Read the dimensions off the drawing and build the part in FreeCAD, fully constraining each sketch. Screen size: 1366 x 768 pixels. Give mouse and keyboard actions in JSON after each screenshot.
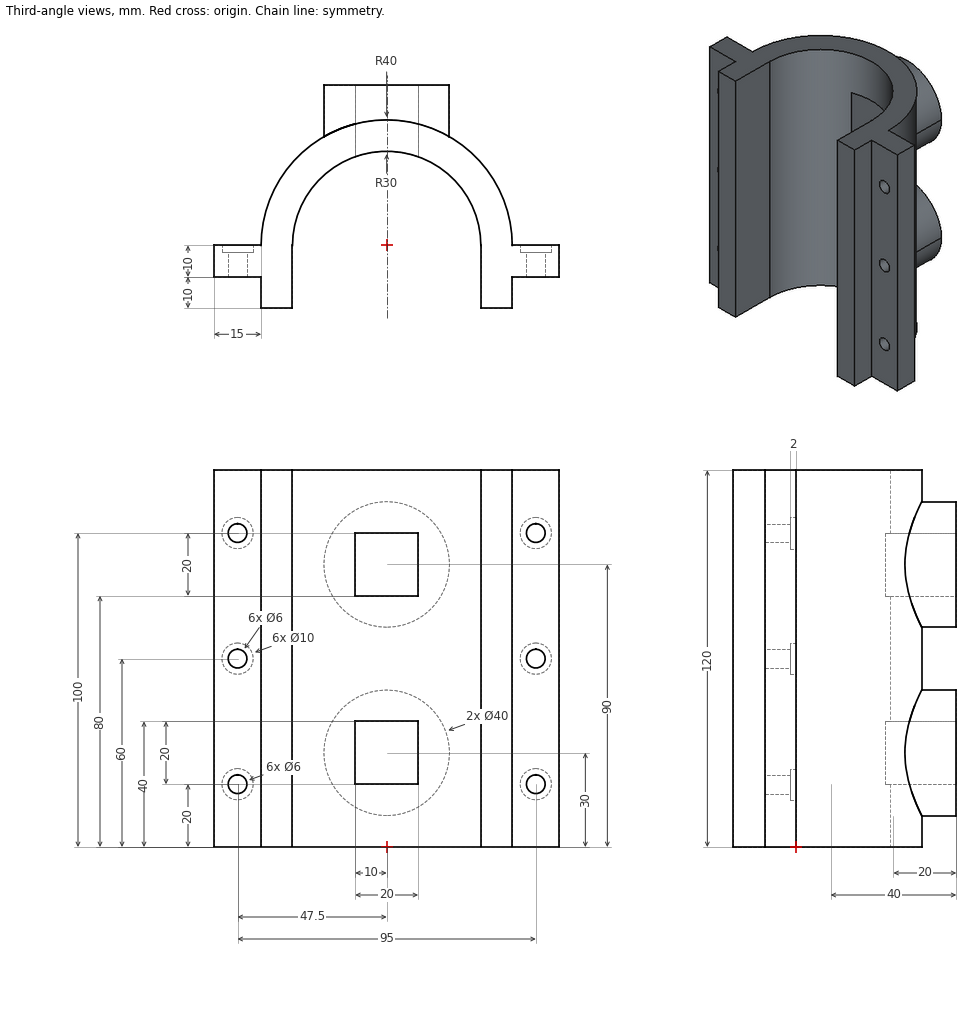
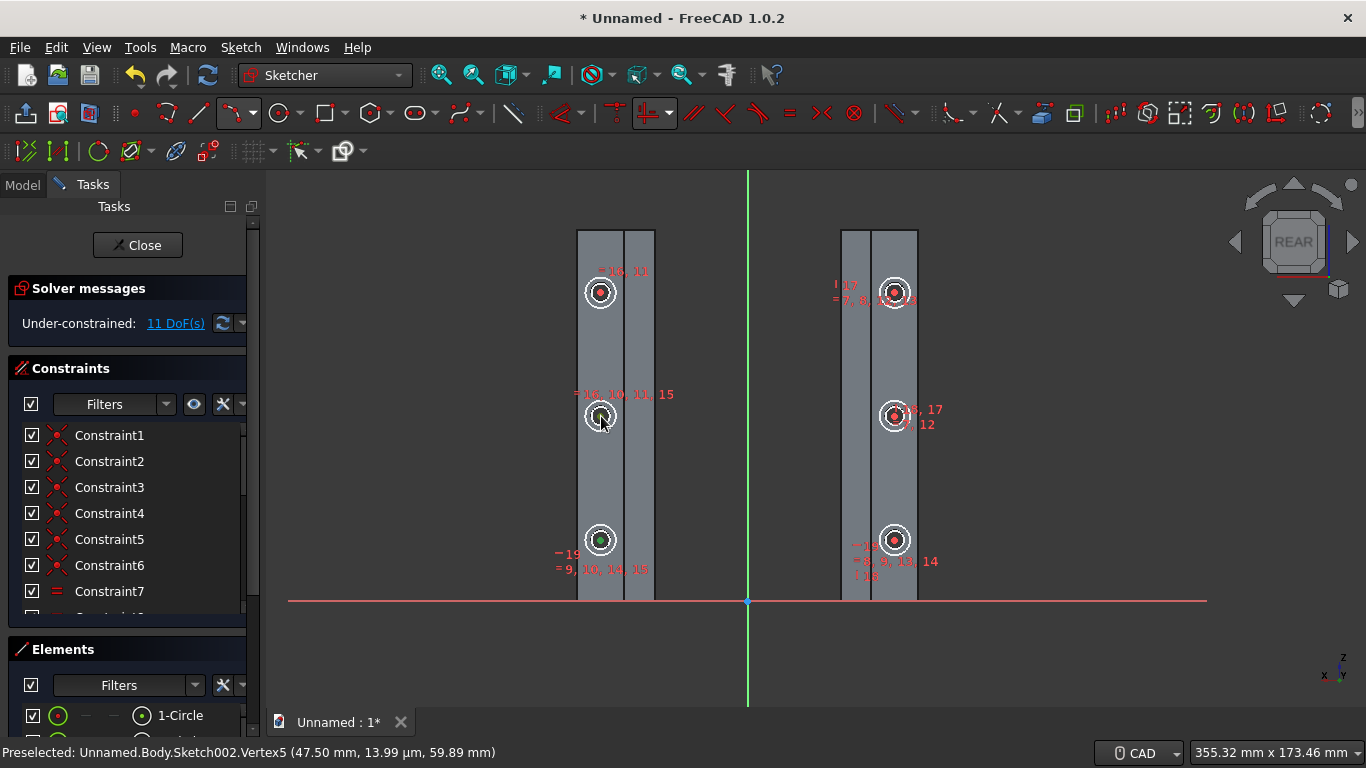
{"action": "left_click", "coordinate": [672, 114]}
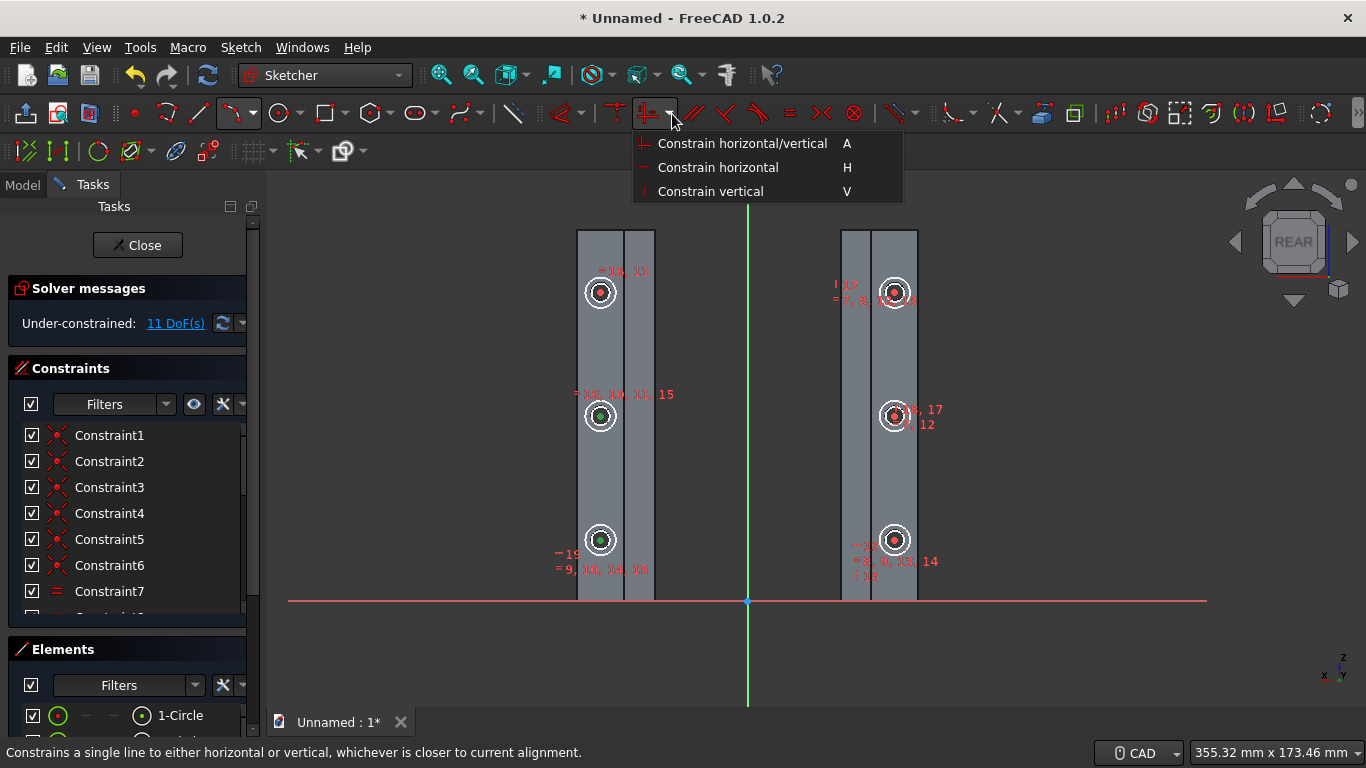
{"action": "left_click", "coordinate": [768, 191]}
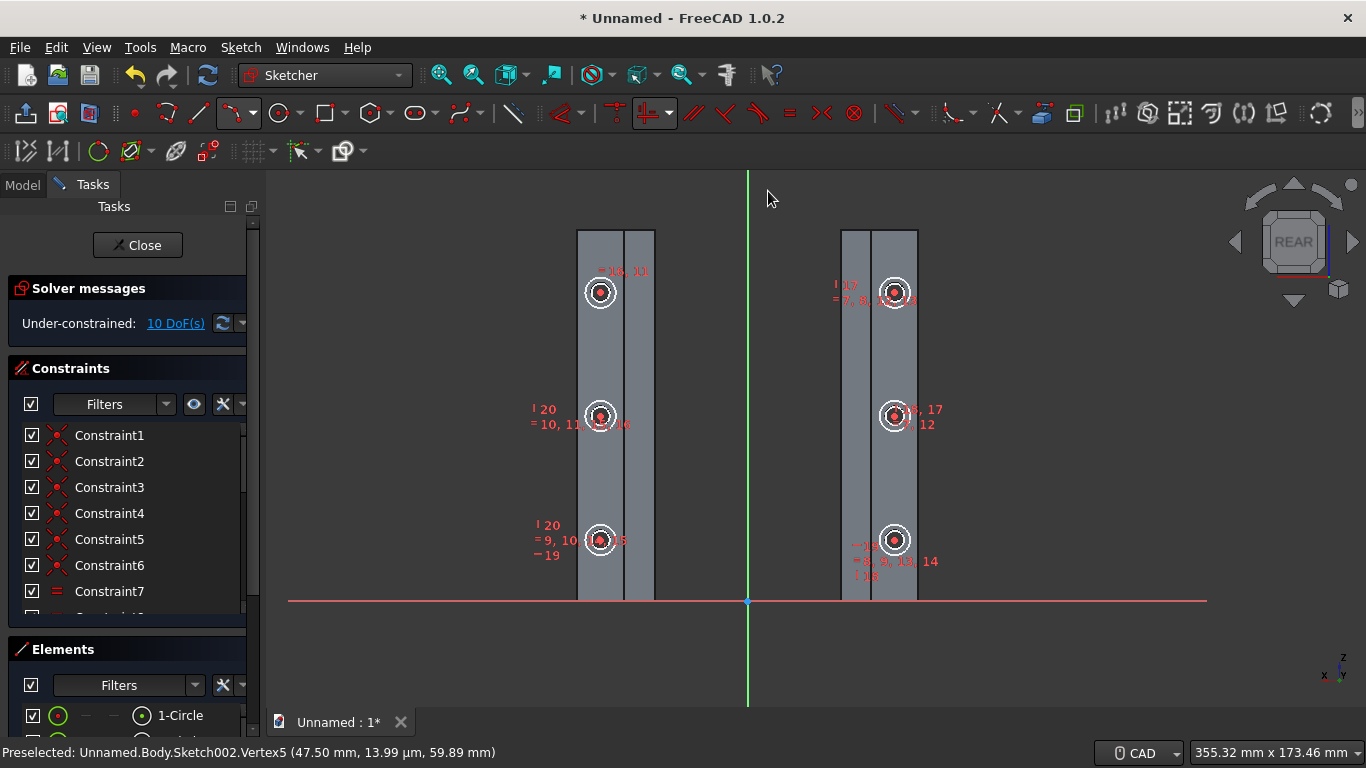
{"action": "left_click", "coordinate": [895, 416]}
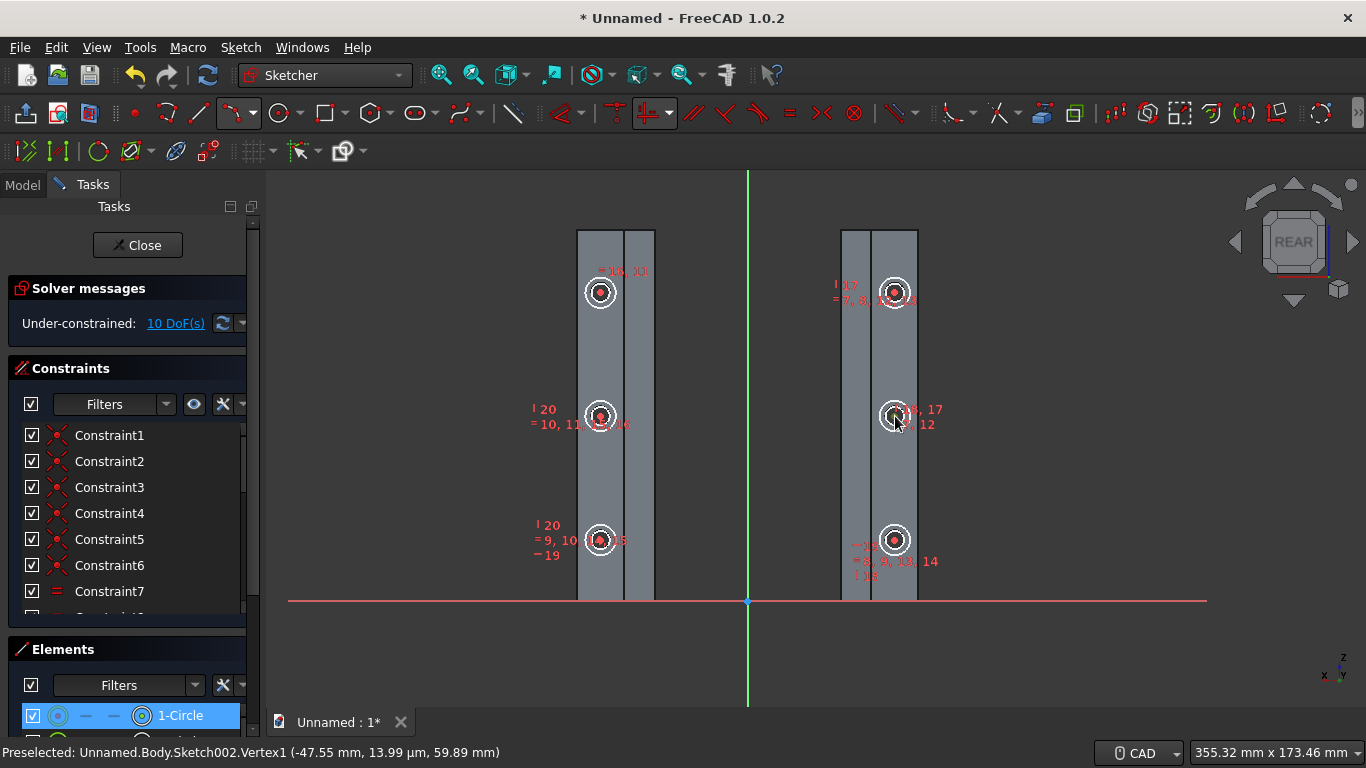
{"action": "scroll", "coordinate": [601, 416], "scroll_direction": "up", "scroll_amount": 4}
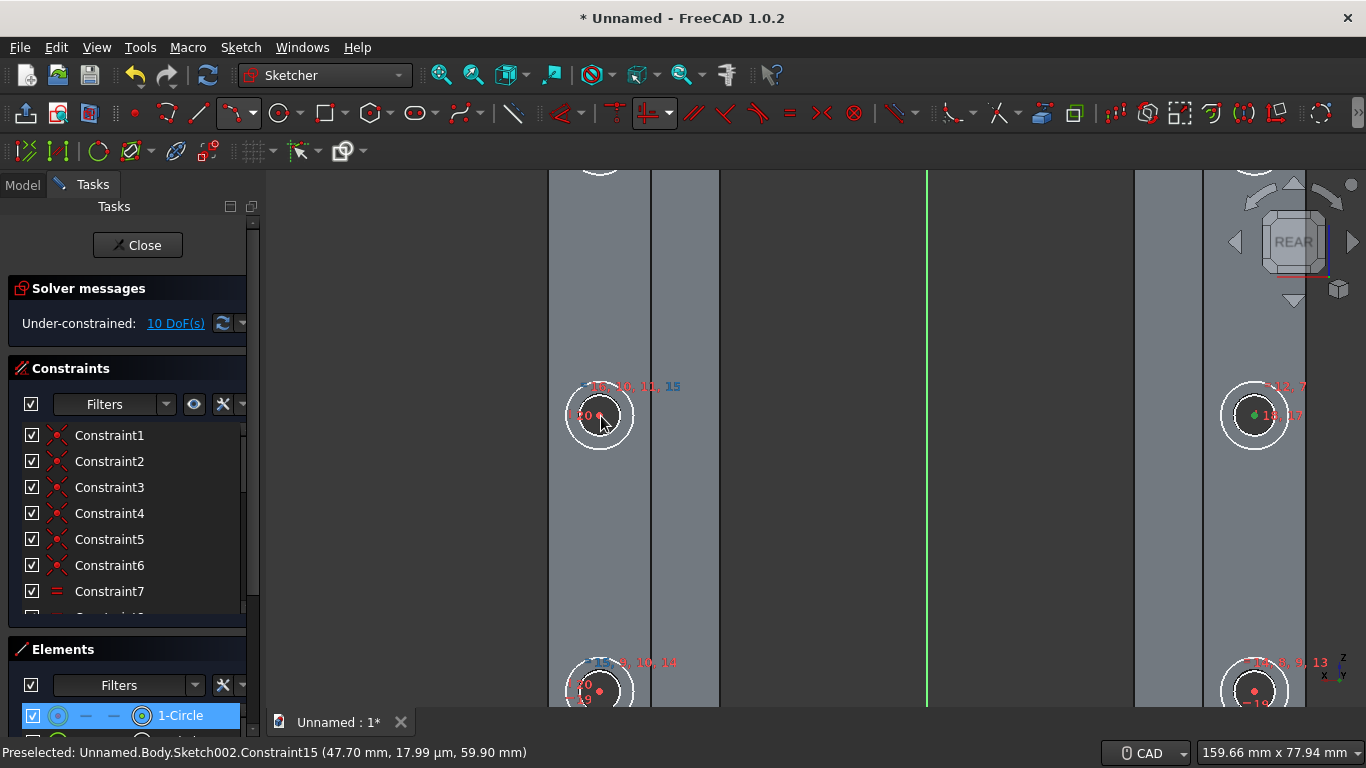
{"action": "left_click", "coordinate": [600, 416]}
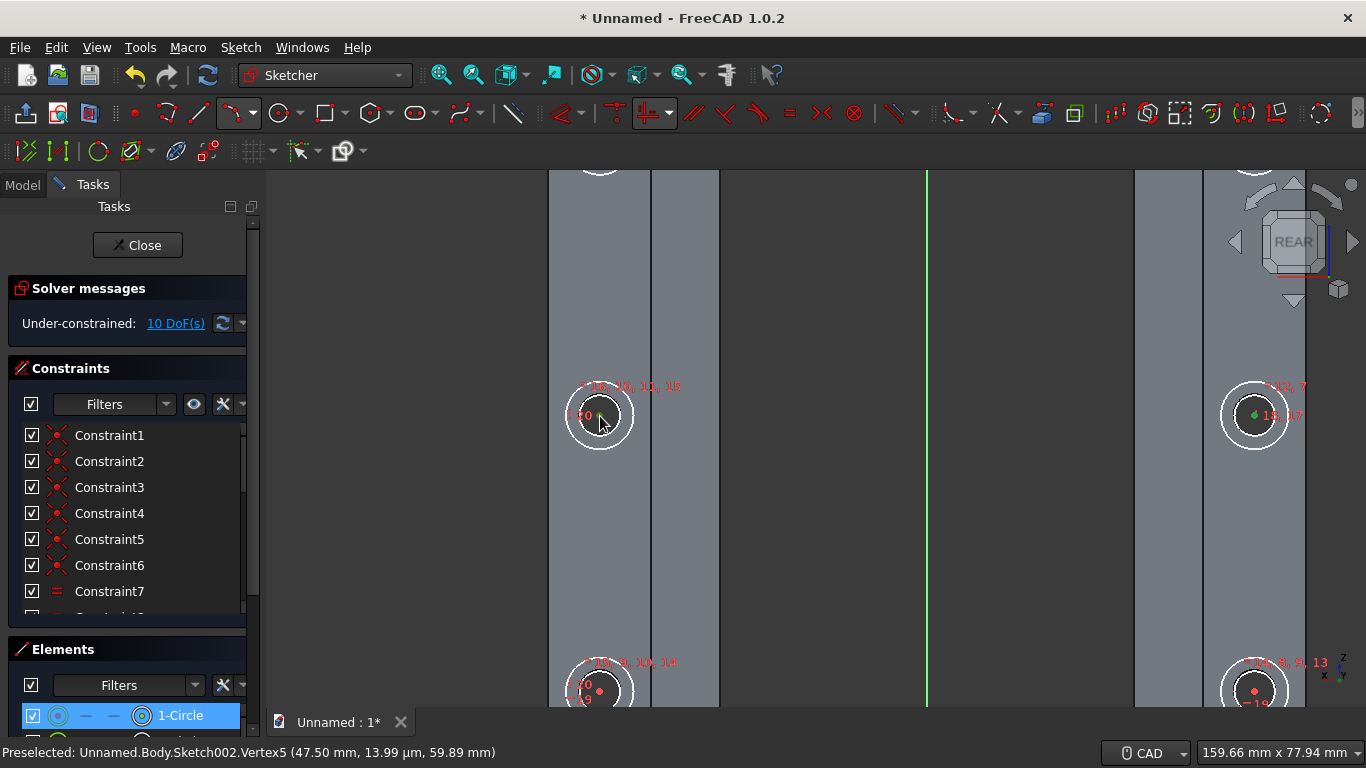
{"action": "left_click", "coordinate": [672, 114]}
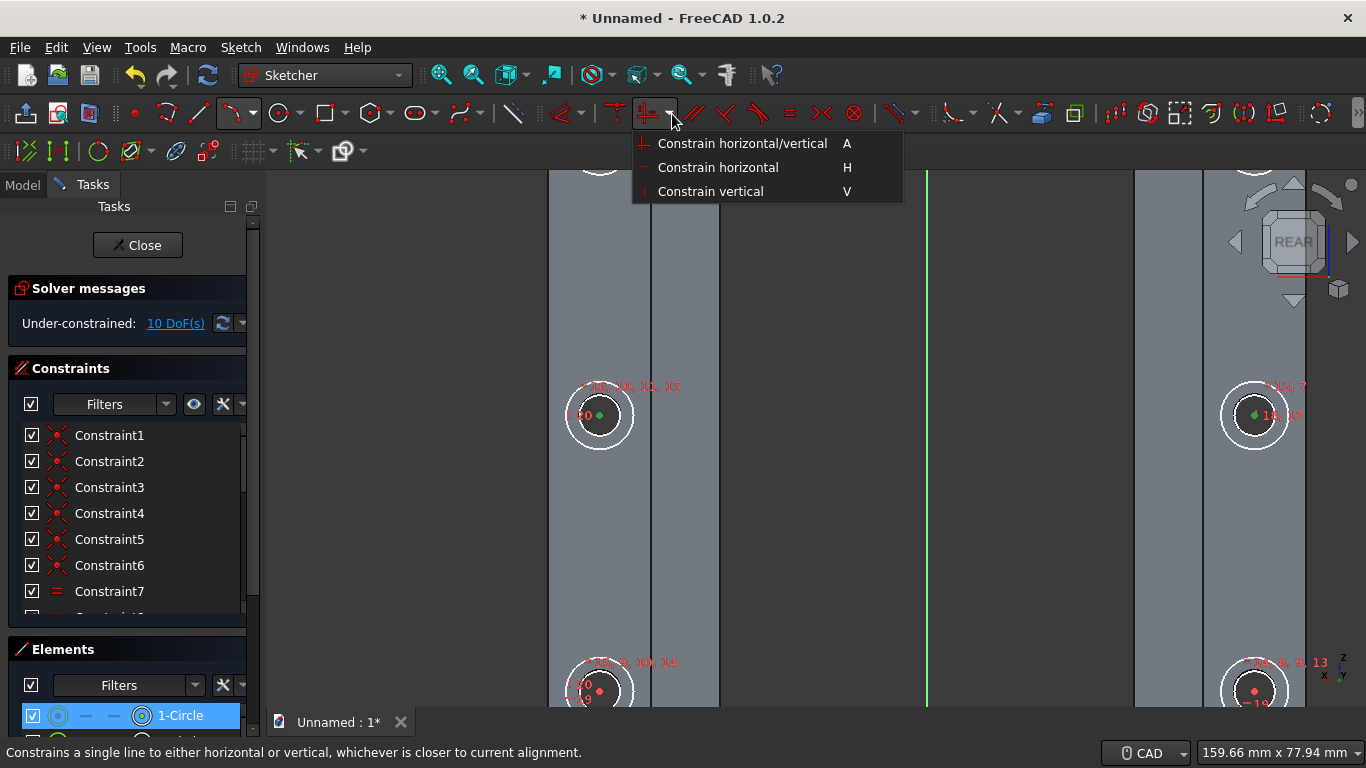
{"action": "left_click", "coordinate": [768, 167]}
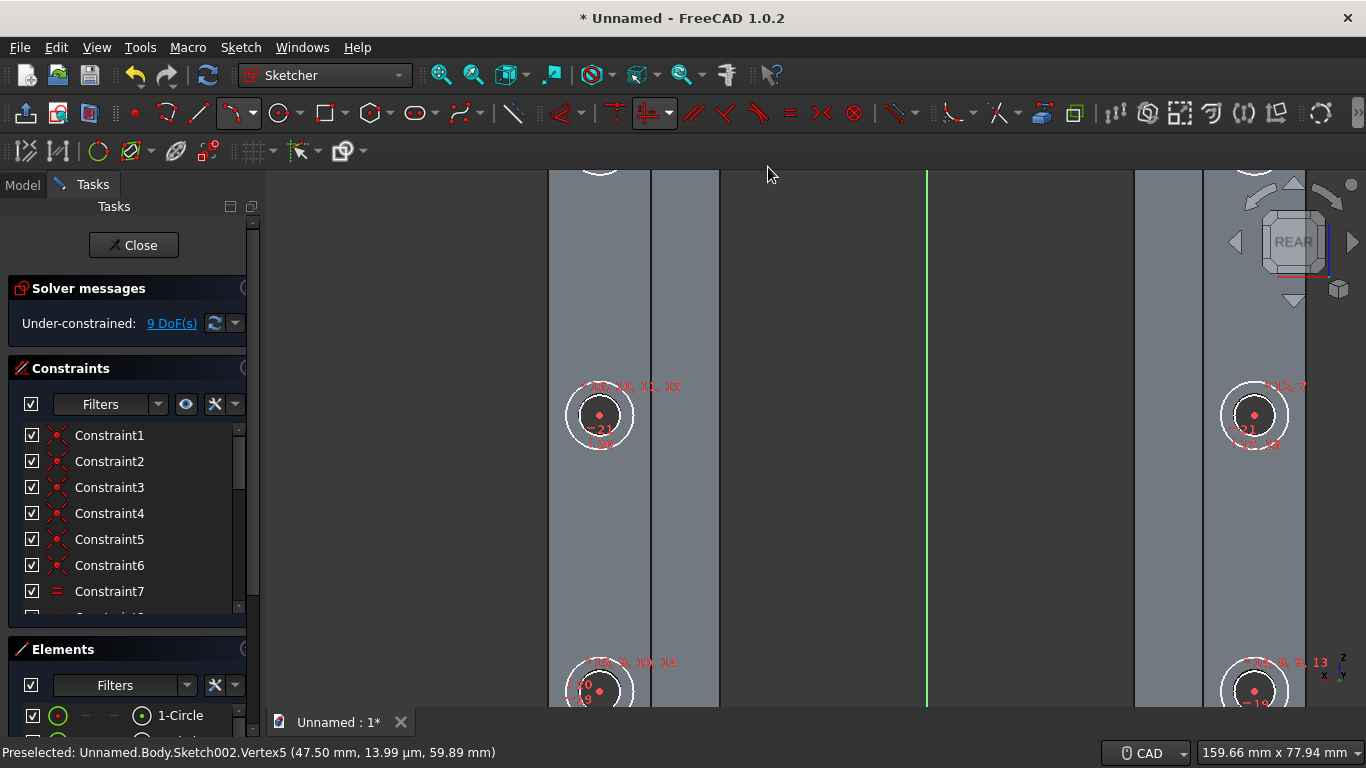
{"action": "left_click", "coordinate": [600, 416]}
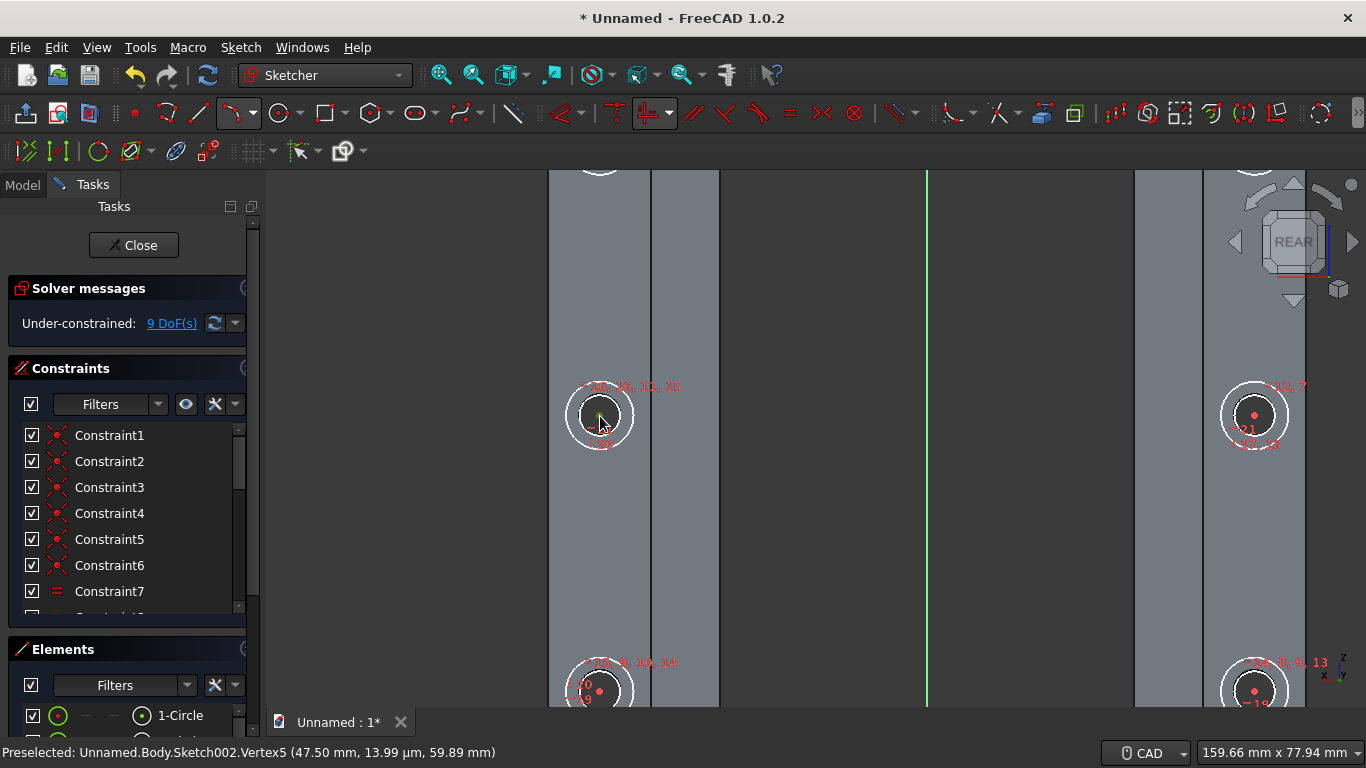
{"action": "scroll", "coordinate": [601, 416], "scroll_direction": "down", "scroll_amount": 4}